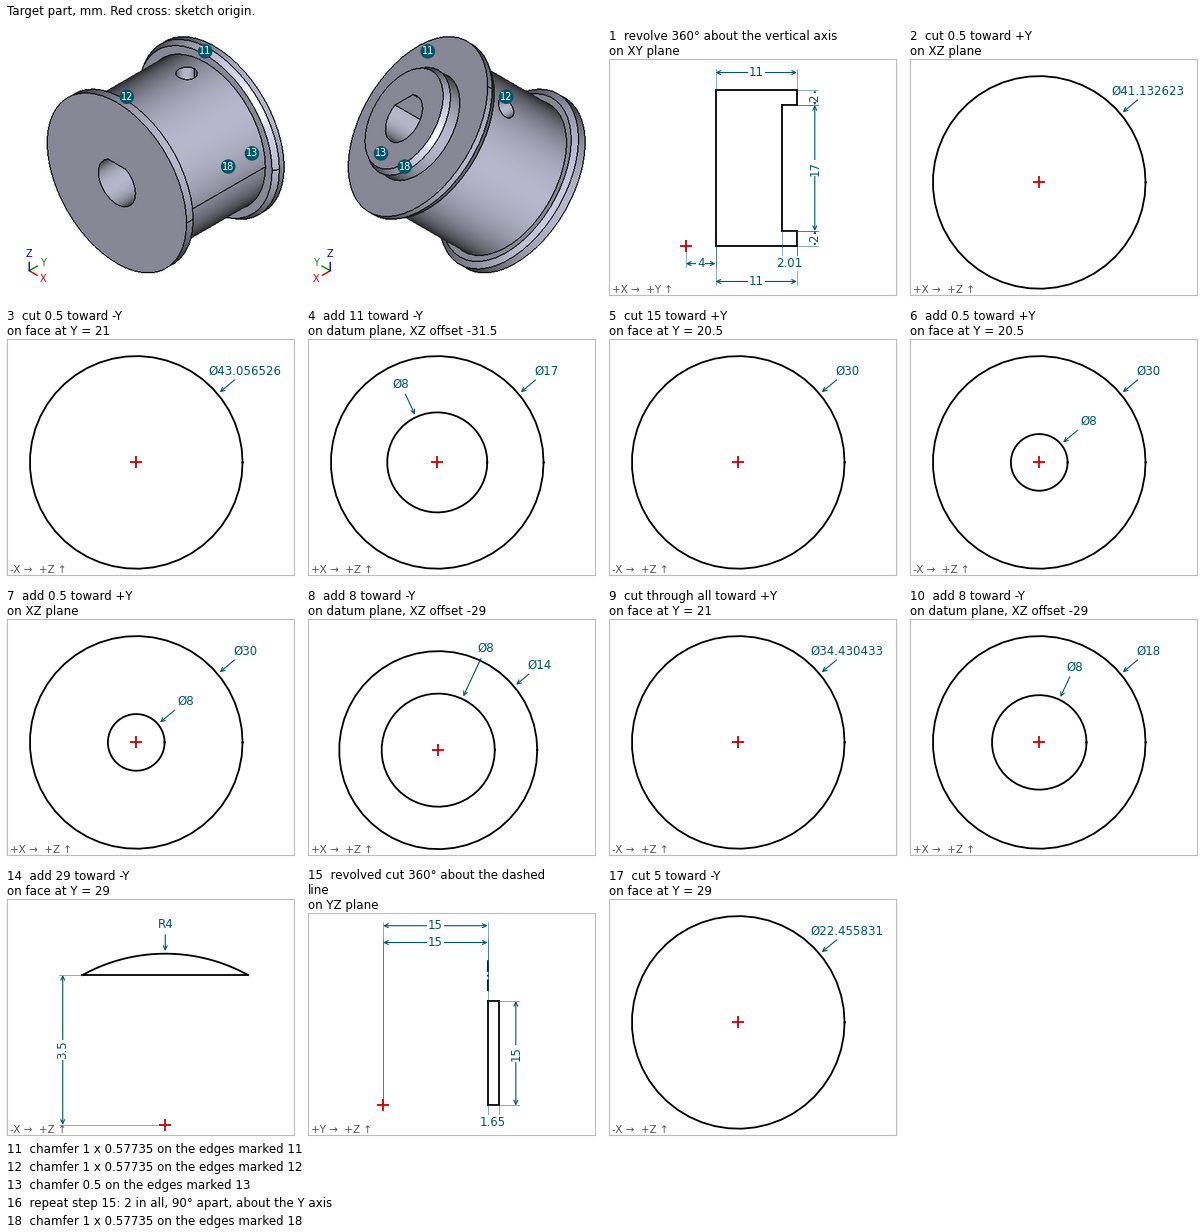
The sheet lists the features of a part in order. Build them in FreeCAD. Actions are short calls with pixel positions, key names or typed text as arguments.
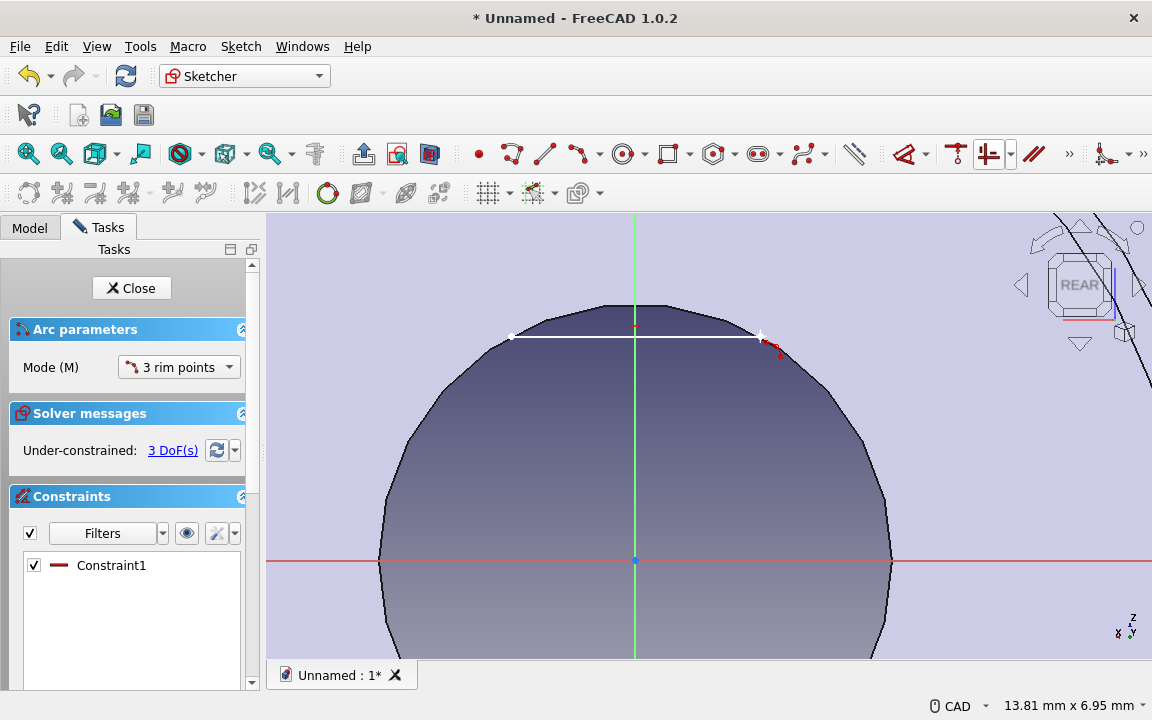
click(760, 337)
click(511, 337)
click(661, 306)
key(Escape)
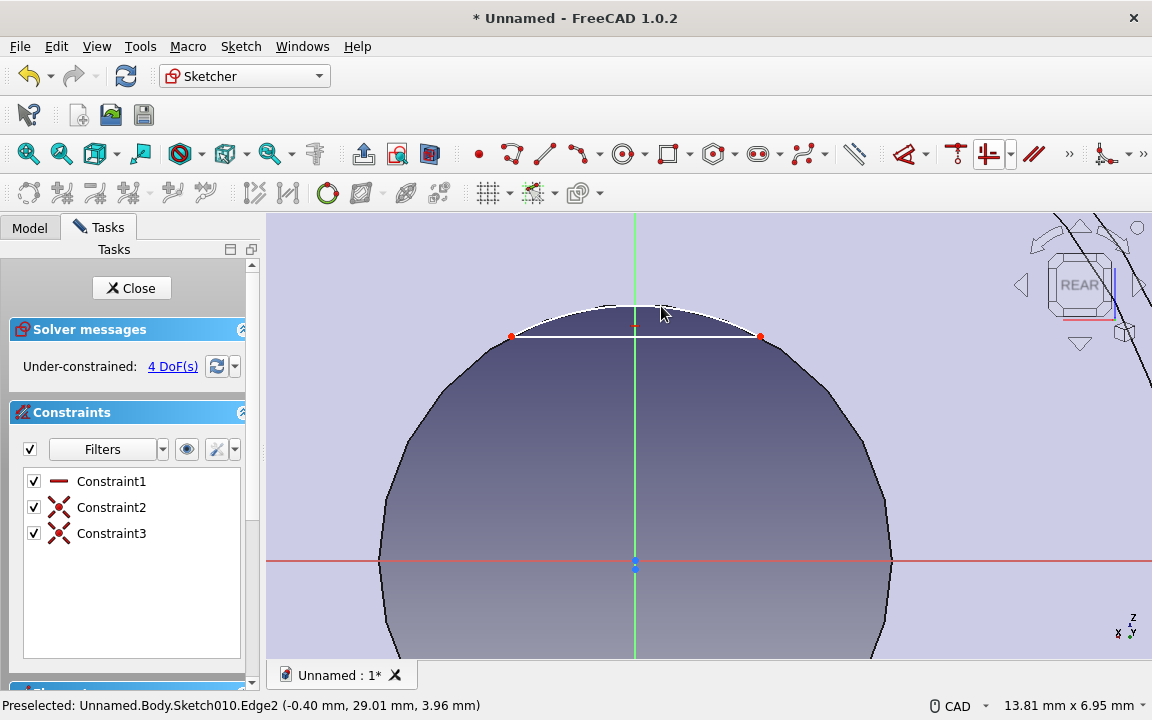
drag(625, 551, 645, 580)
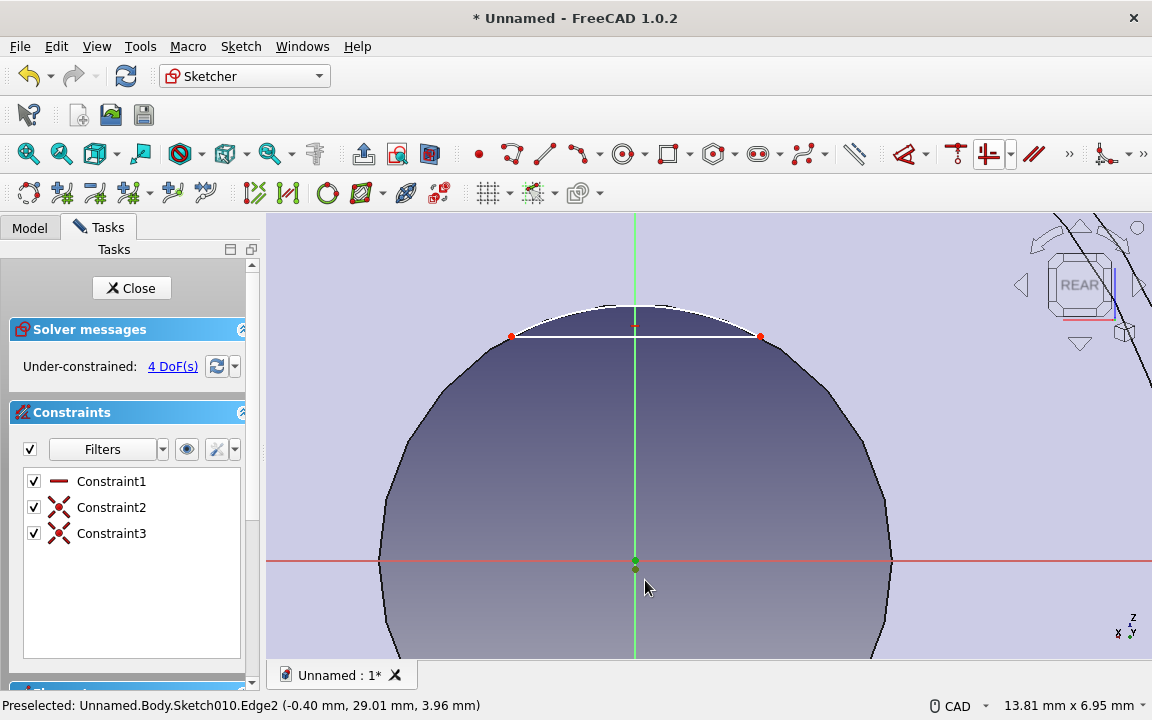
click(956, 154)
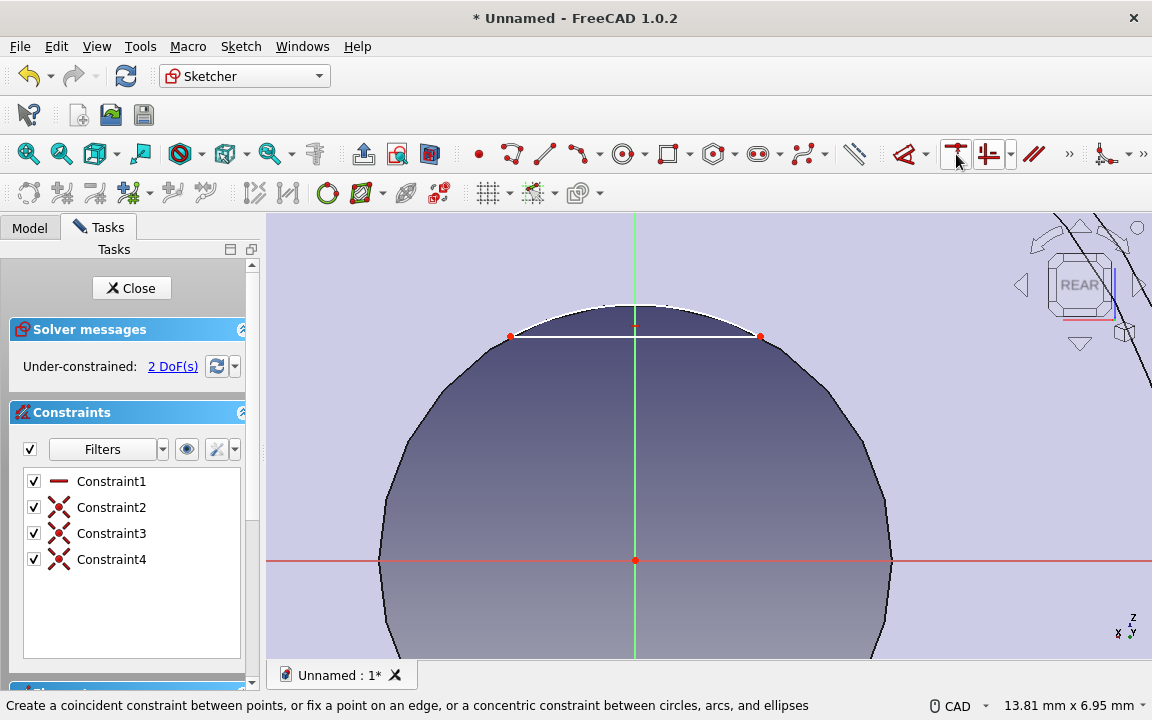
click(904, 154)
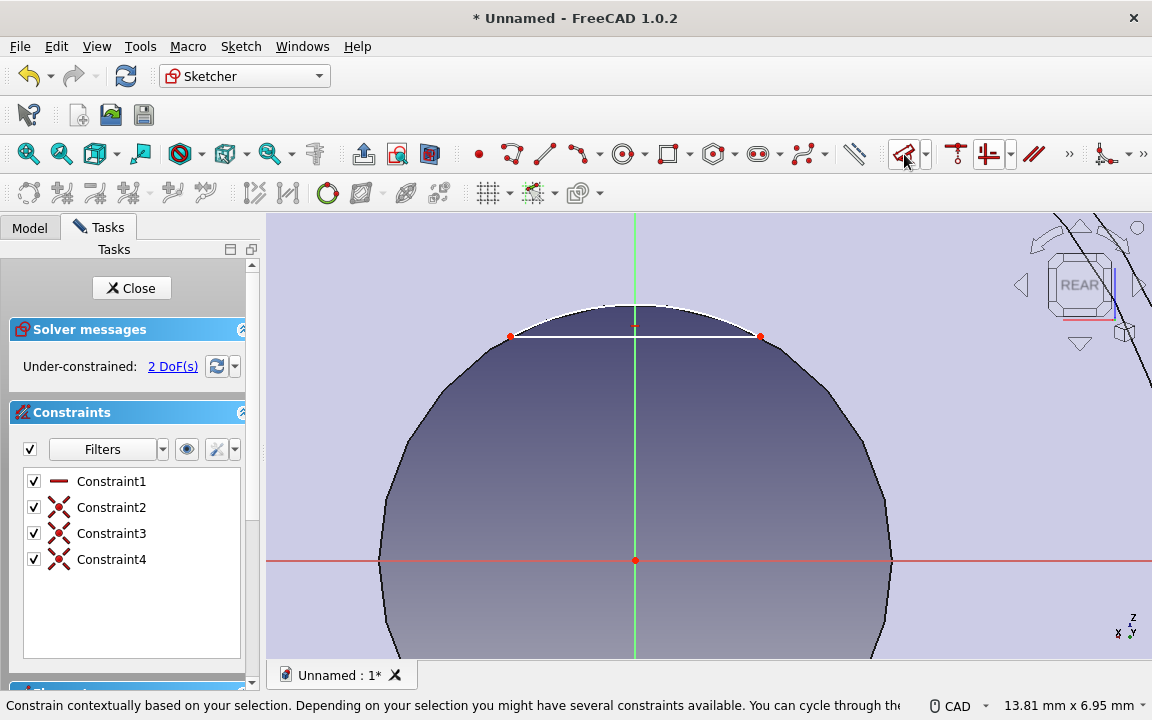
click(687, 310)
click(693, 279)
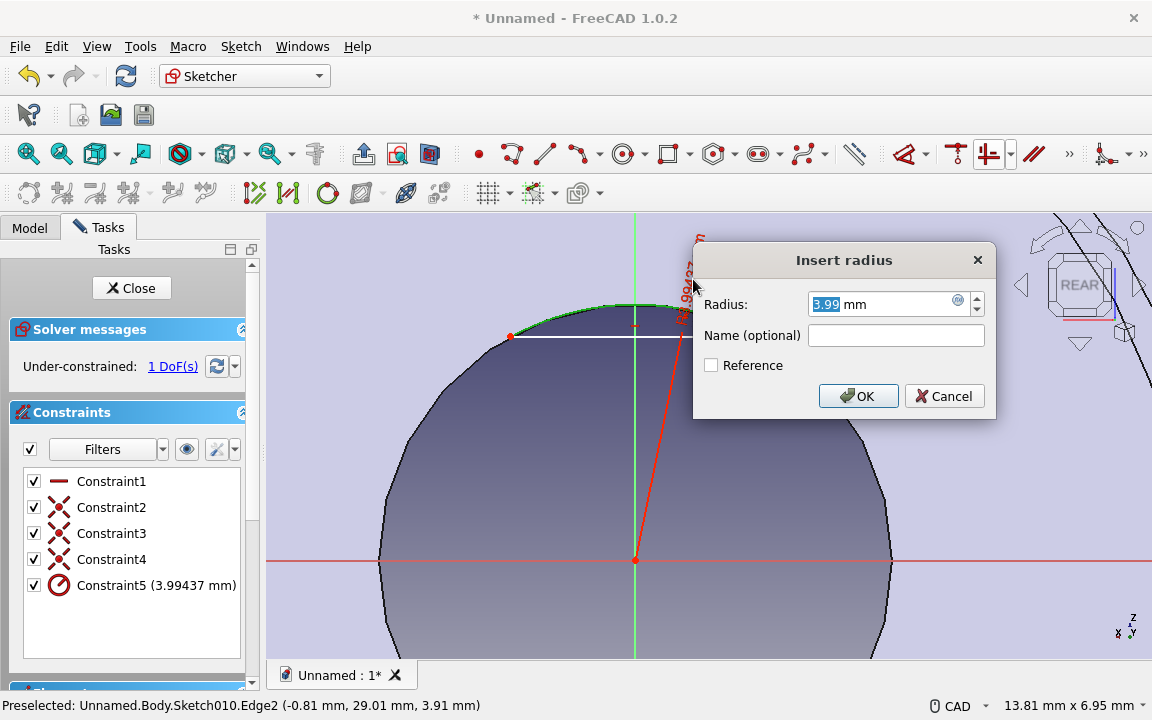
text(4)
key(Return)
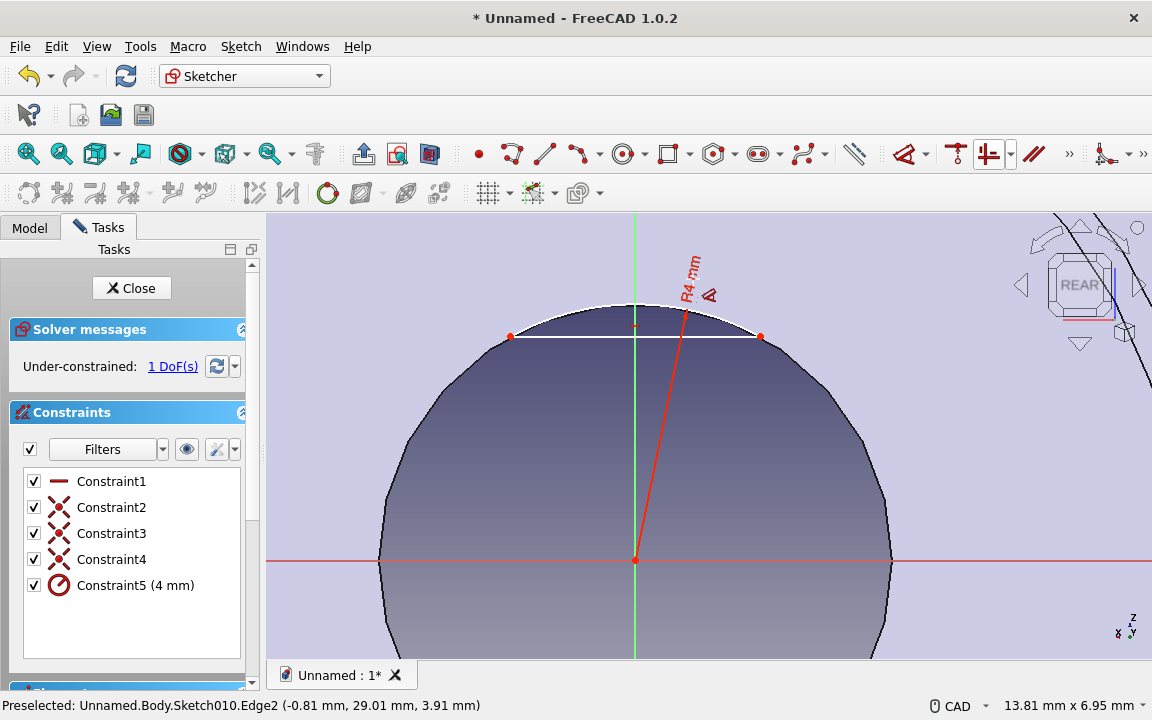
click(511, 337)
click(477, 449)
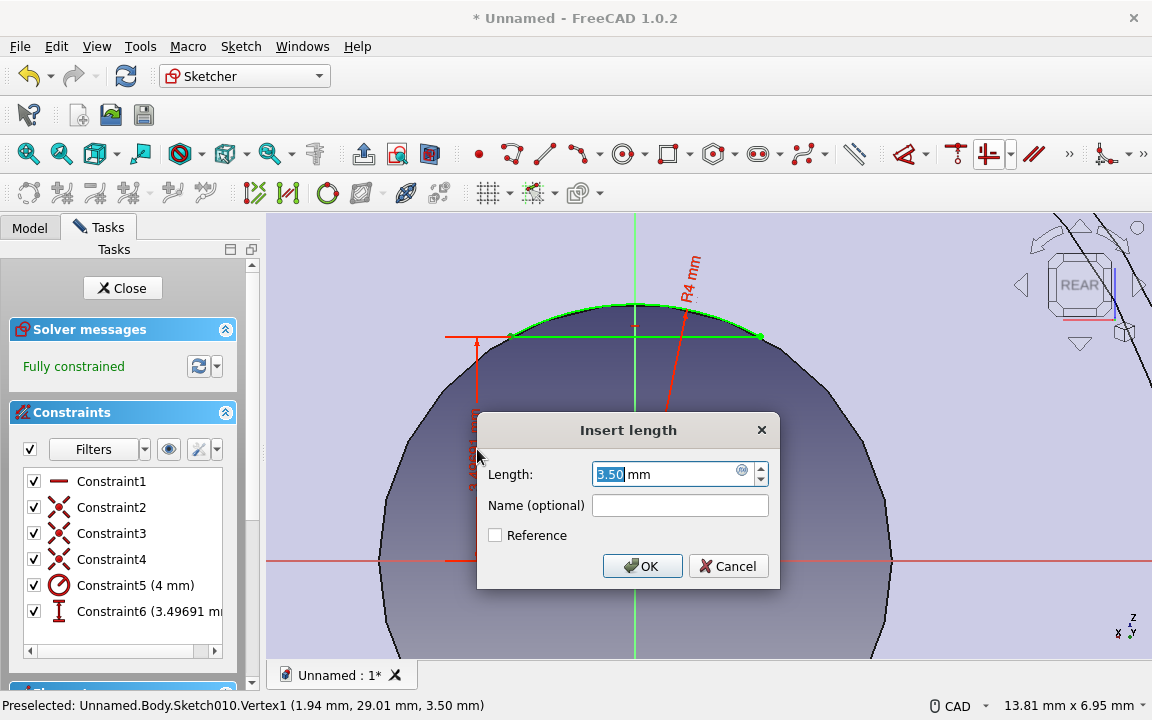
text(3.5)
key(Return)
key(Escape)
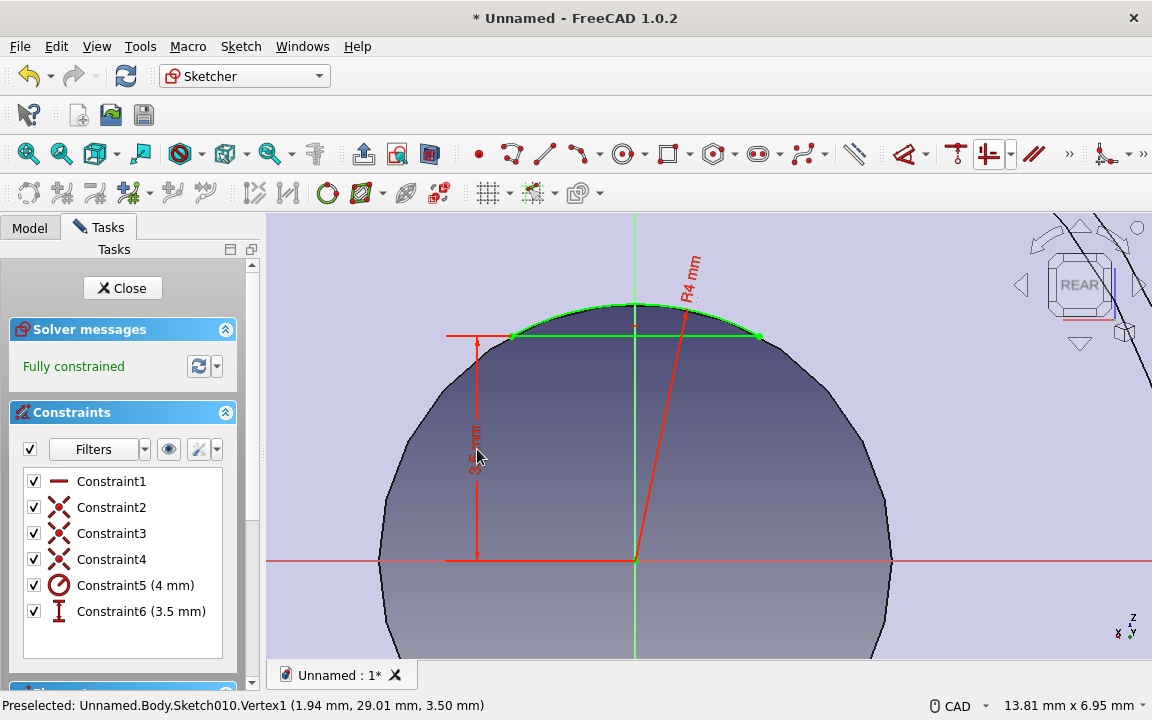
click(123, 288)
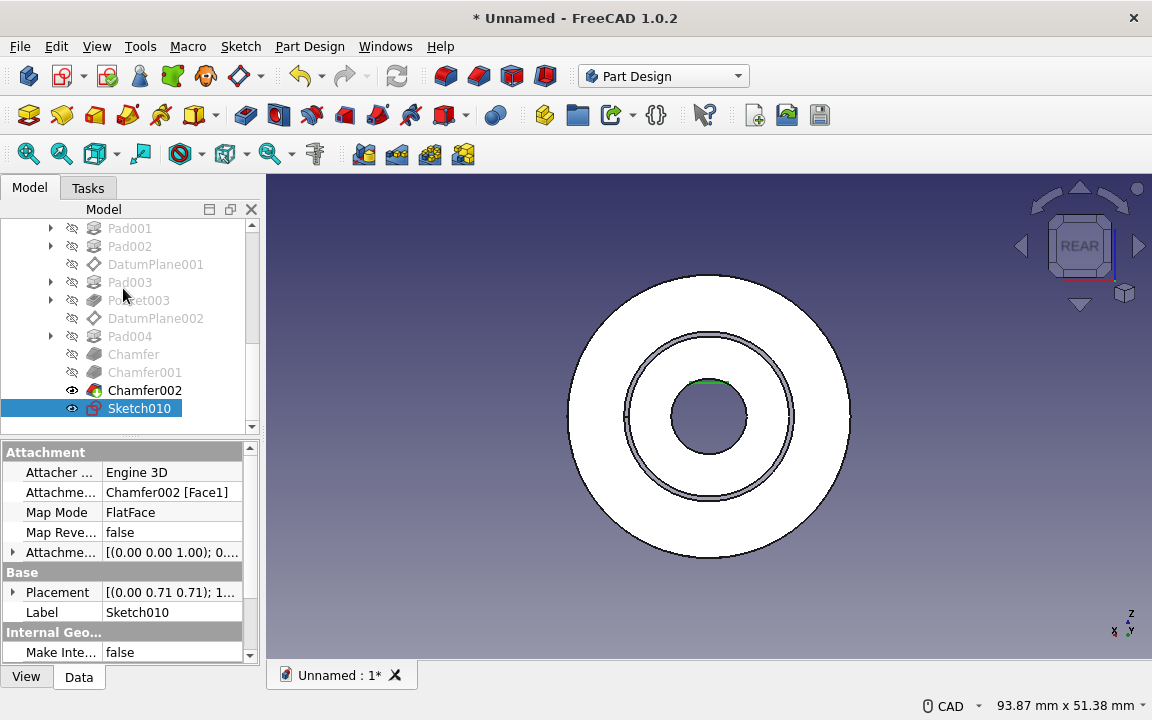
click(29, 116)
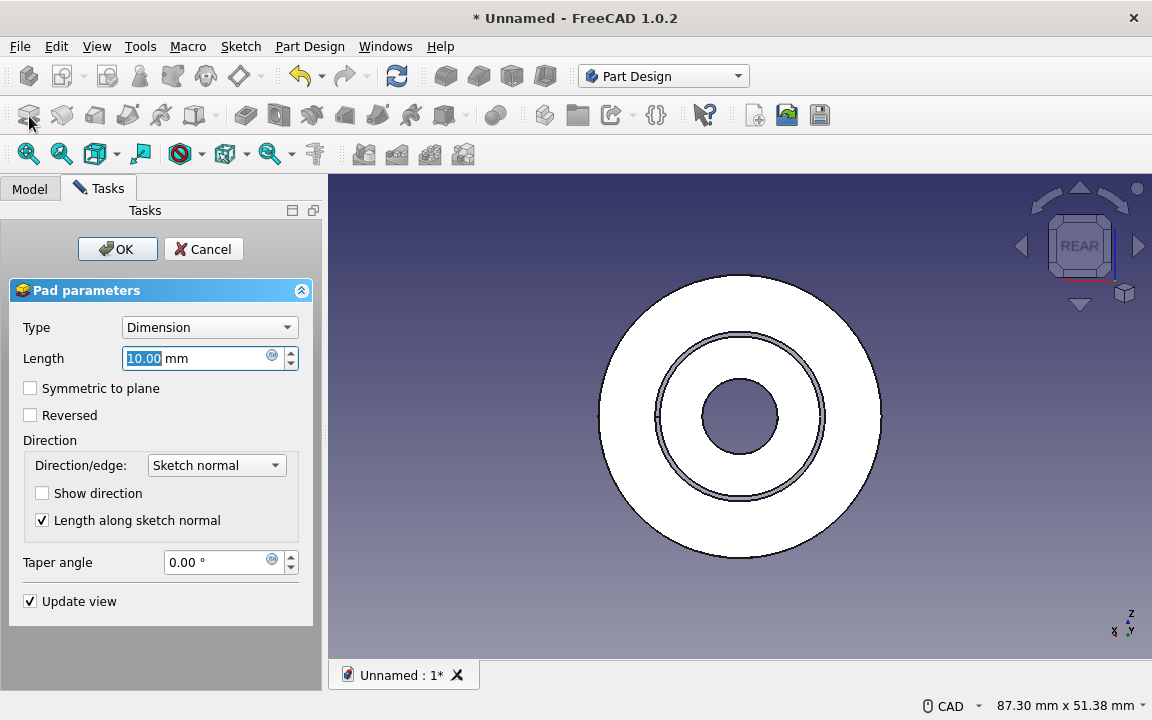
text(29)
key(Tab)